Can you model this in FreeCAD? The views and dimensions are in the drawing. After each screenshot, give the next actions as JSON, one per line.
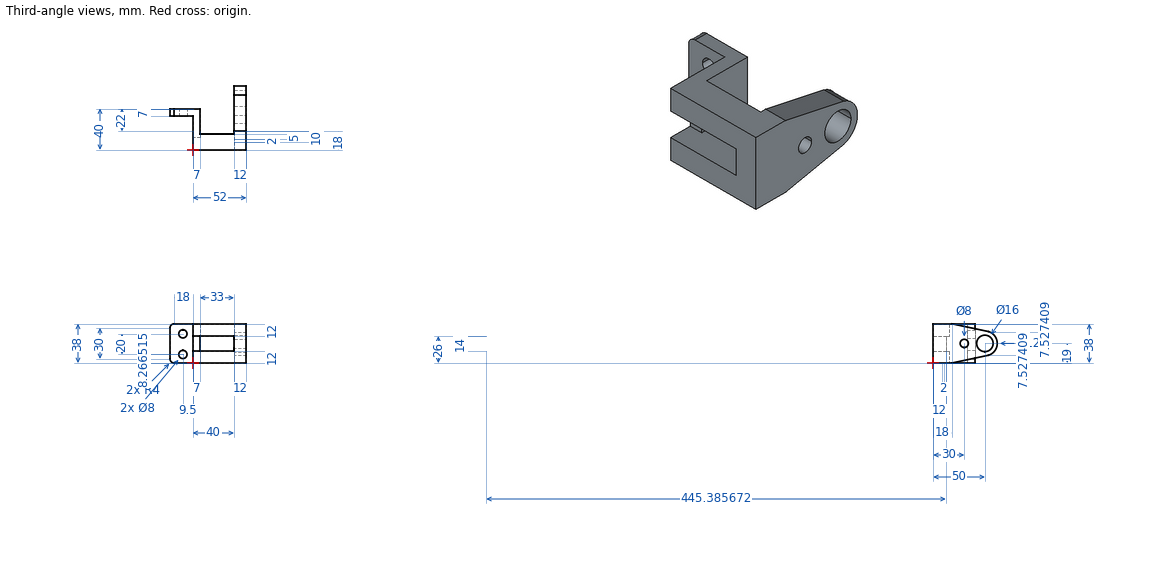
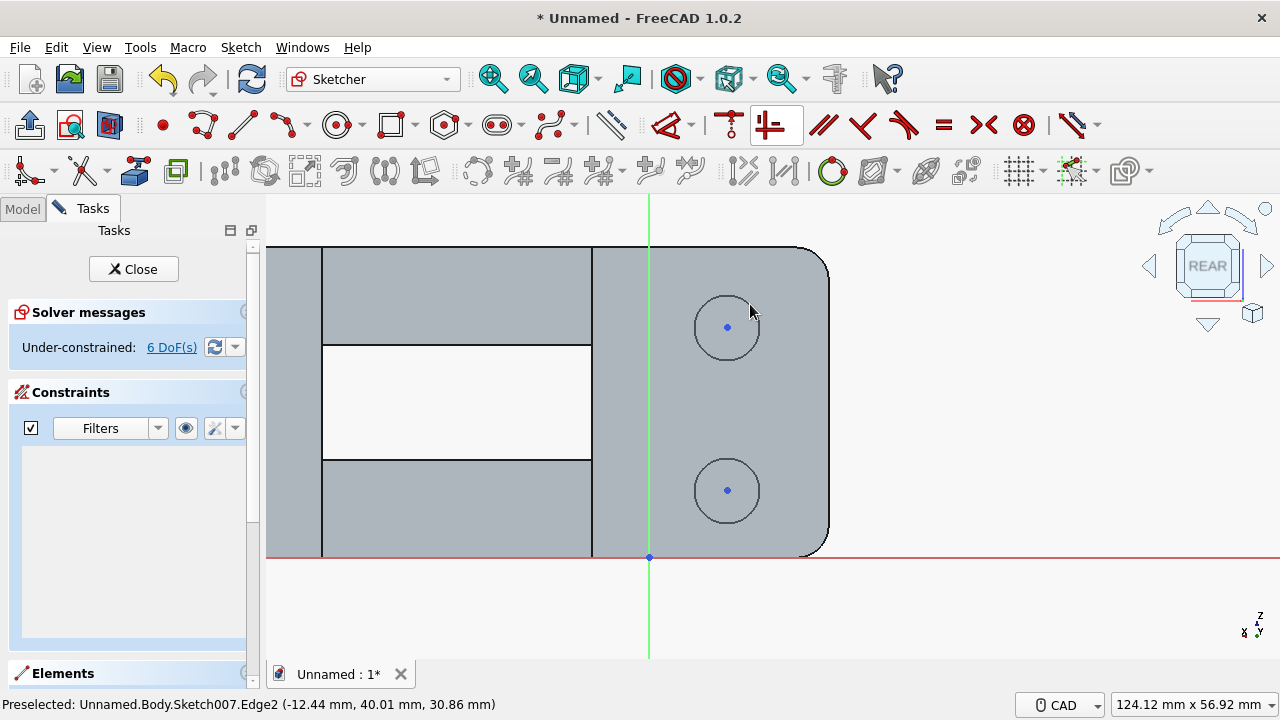
{"action": "left_click", "coordinate": [750, 468]}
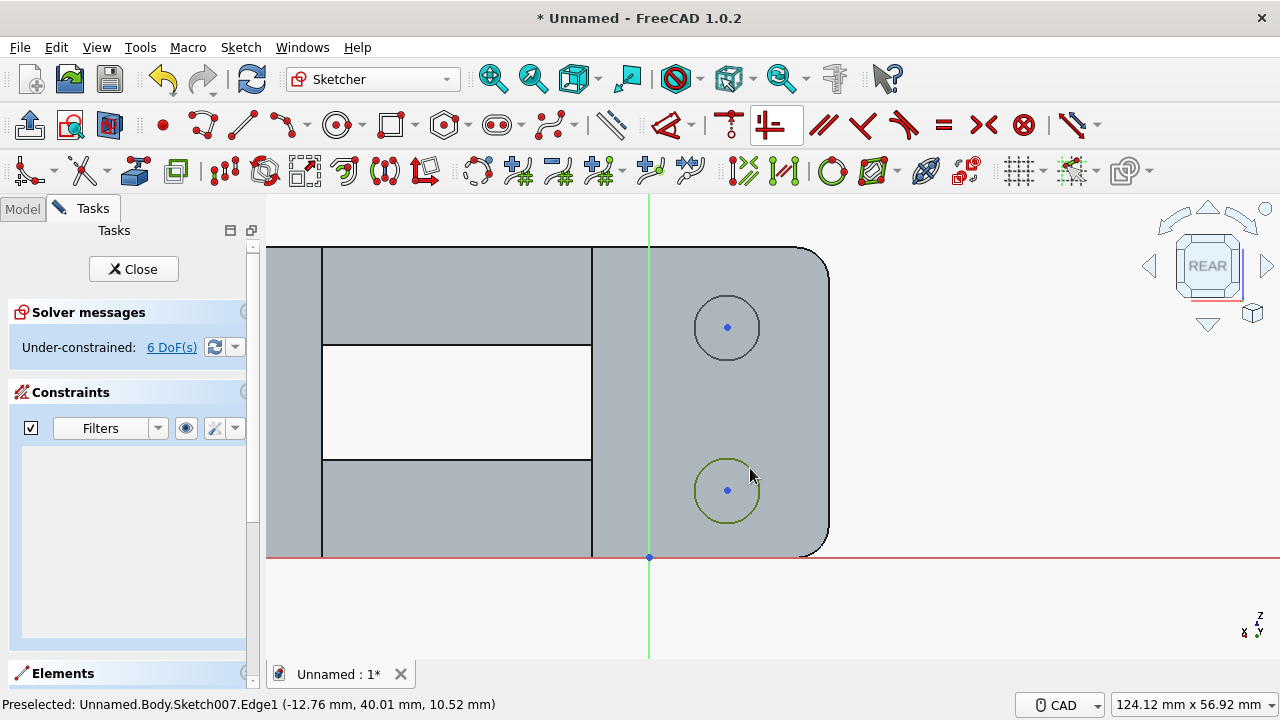
{"action": "left_click", "coordinate": [750, 305]}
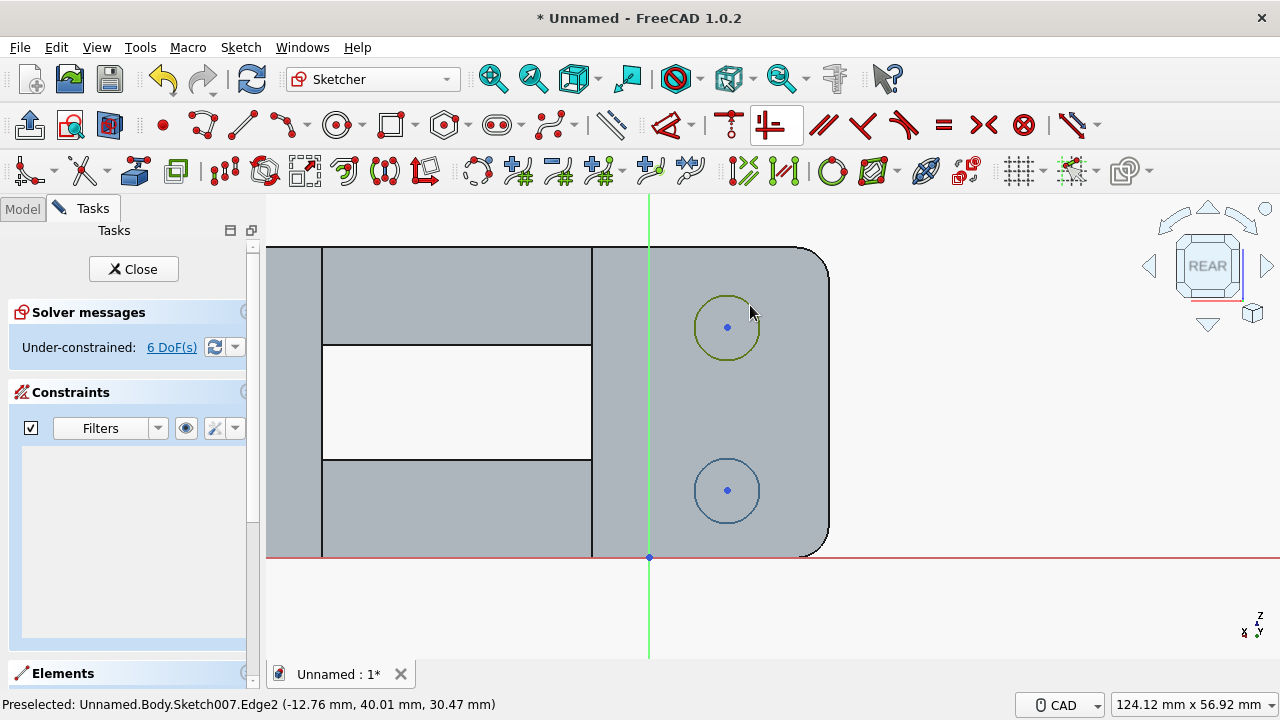
{"action": "left_click", "coordinate": [944, 126]}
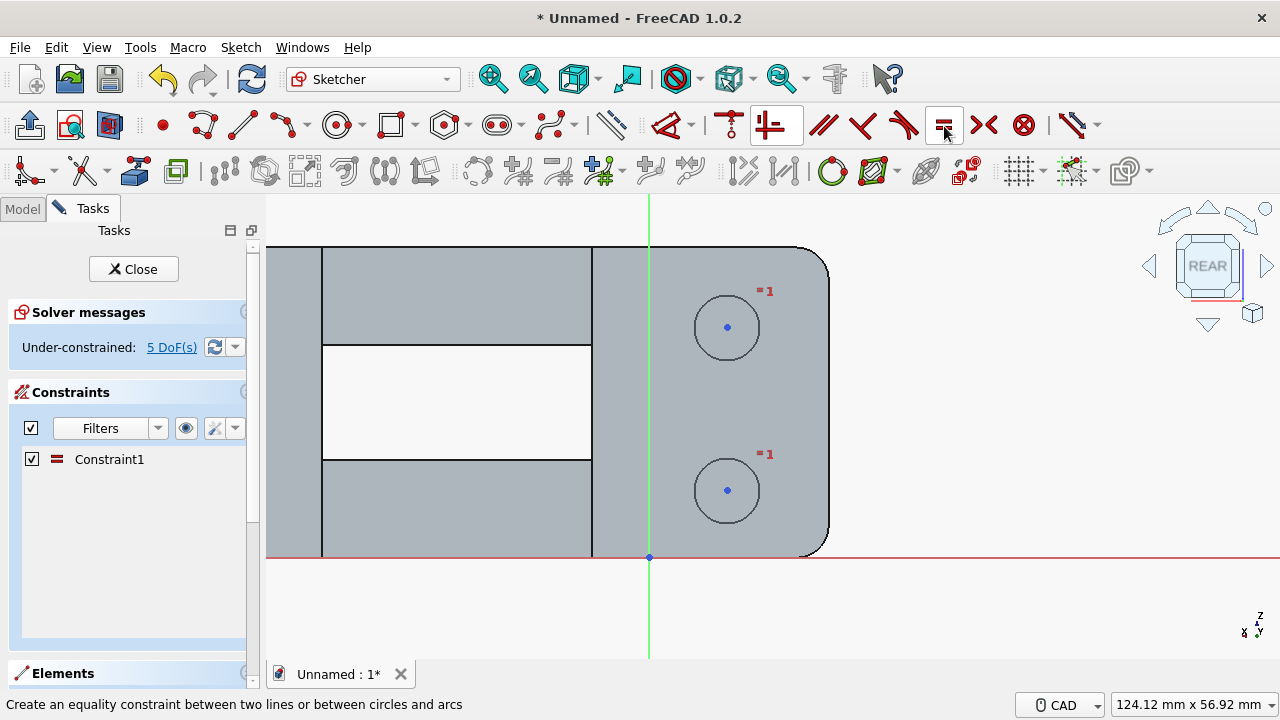
{"action": "left_click", "coordinate": [666, 126]}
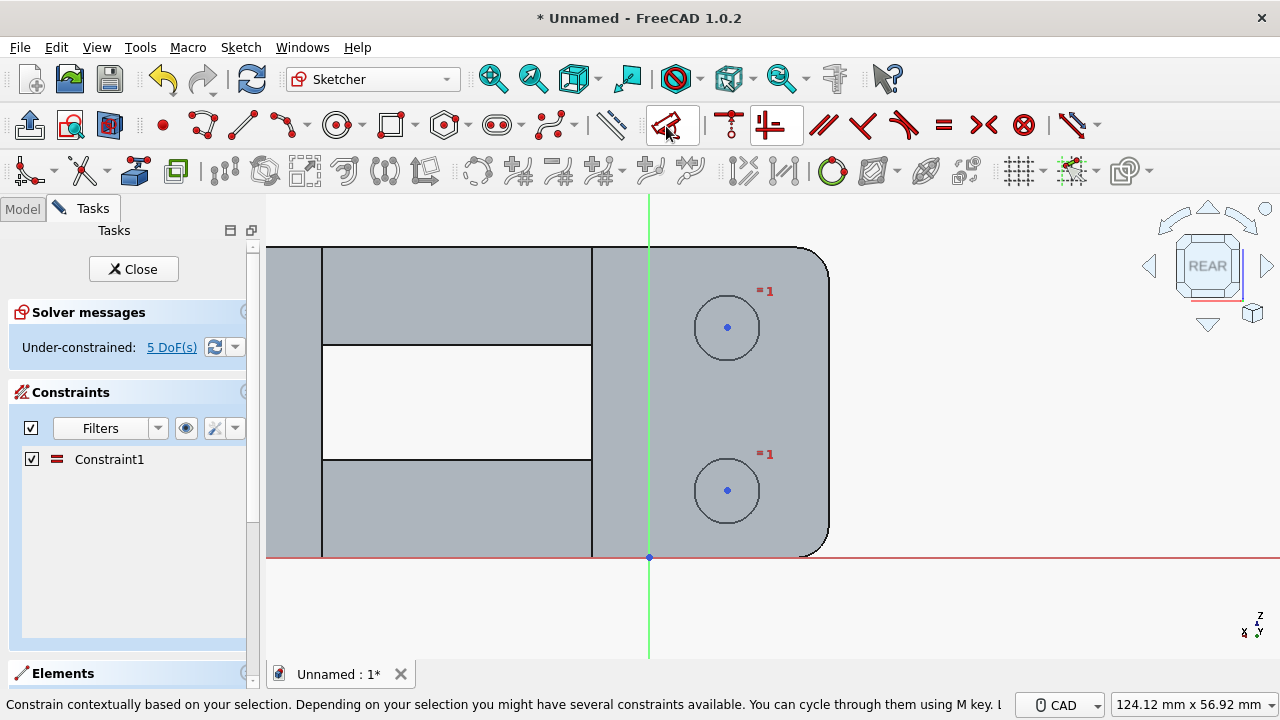
{"action": "left_click", "coordinate": [750, 468]}
{"action": "left_click", "coordinate": [773, 445]}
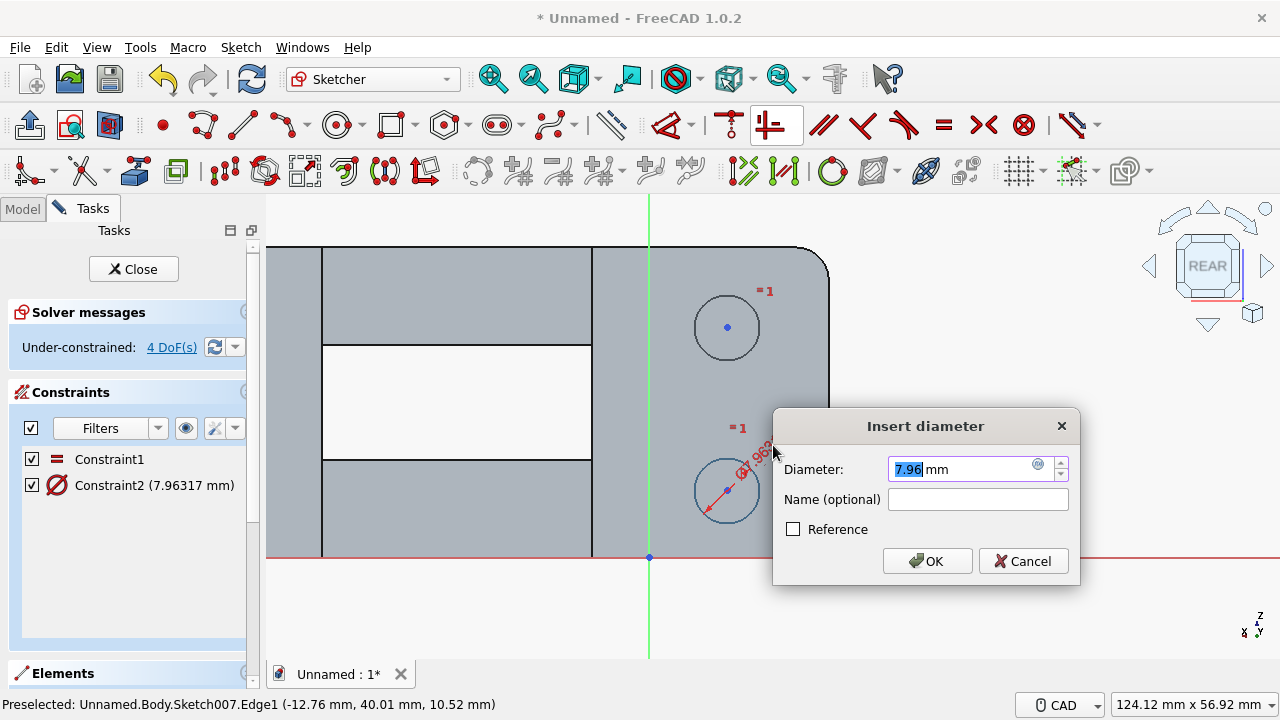
{"action": "type", "text": "8"}
{"action": "key", "text": "Return"}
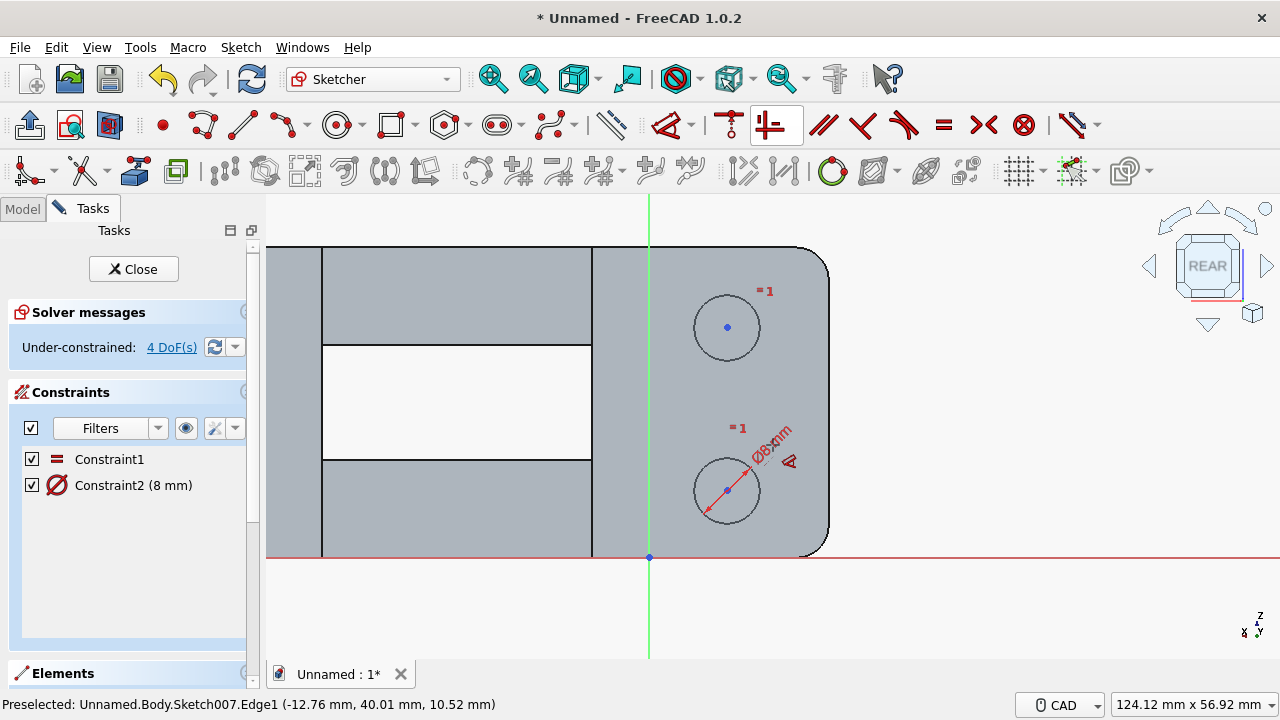
{"action": "left_click", "coordinate": [727, 491]}
{"action": "left_click", "coordinate": [688, 592]}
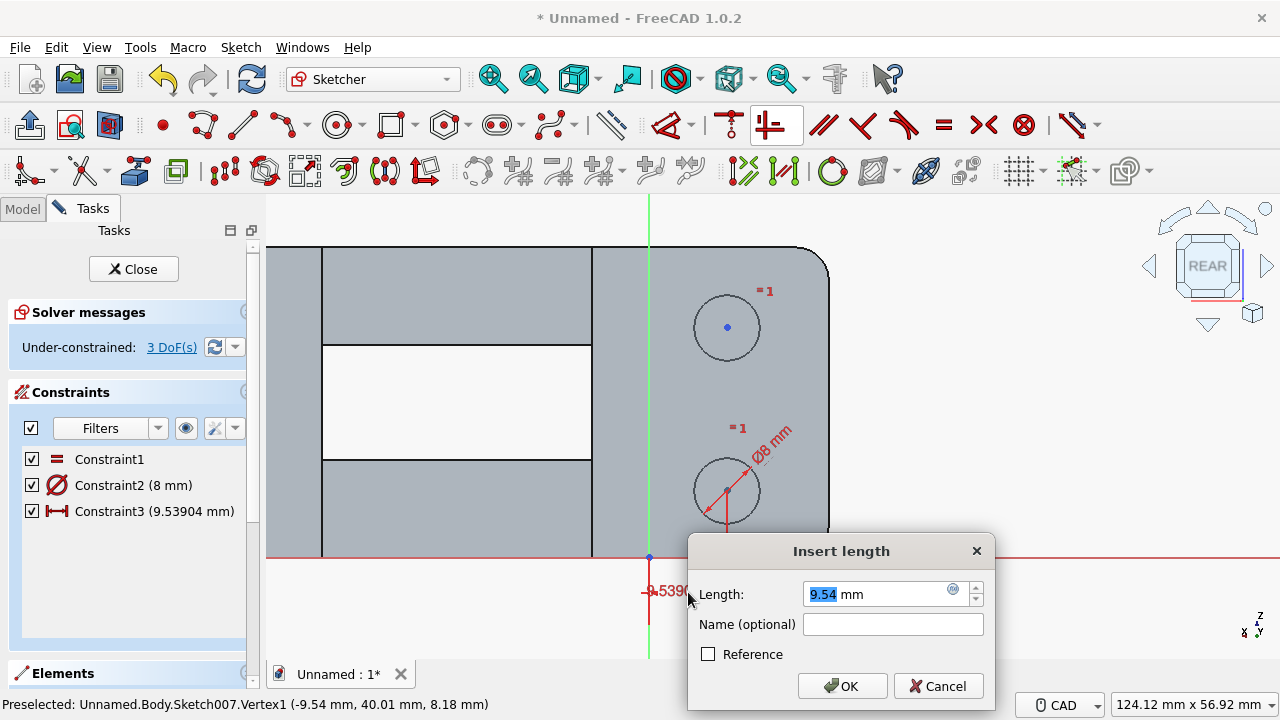
{"action": "type", "text": "9.5"}
{"action": "key", "text": "Return"}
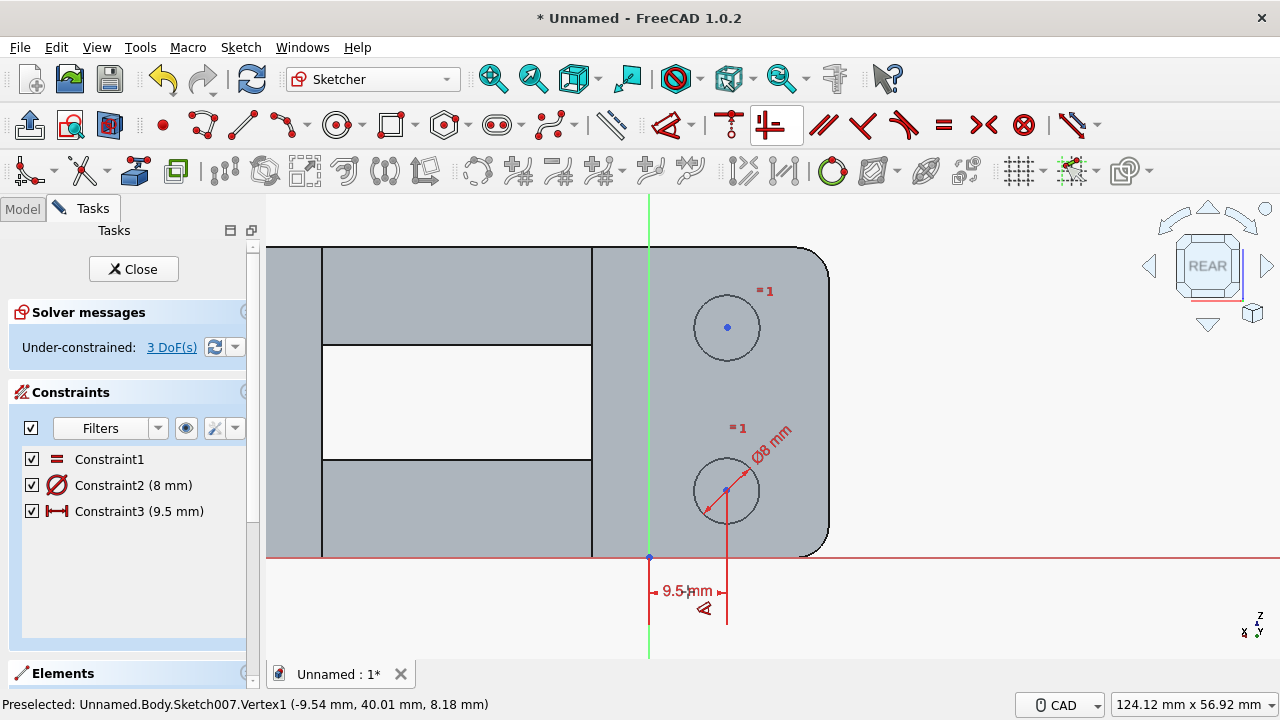
{"action": "left_click", "coordinate": [727, 328]}
{"action": "left_click", "coordinate": [688, 294]}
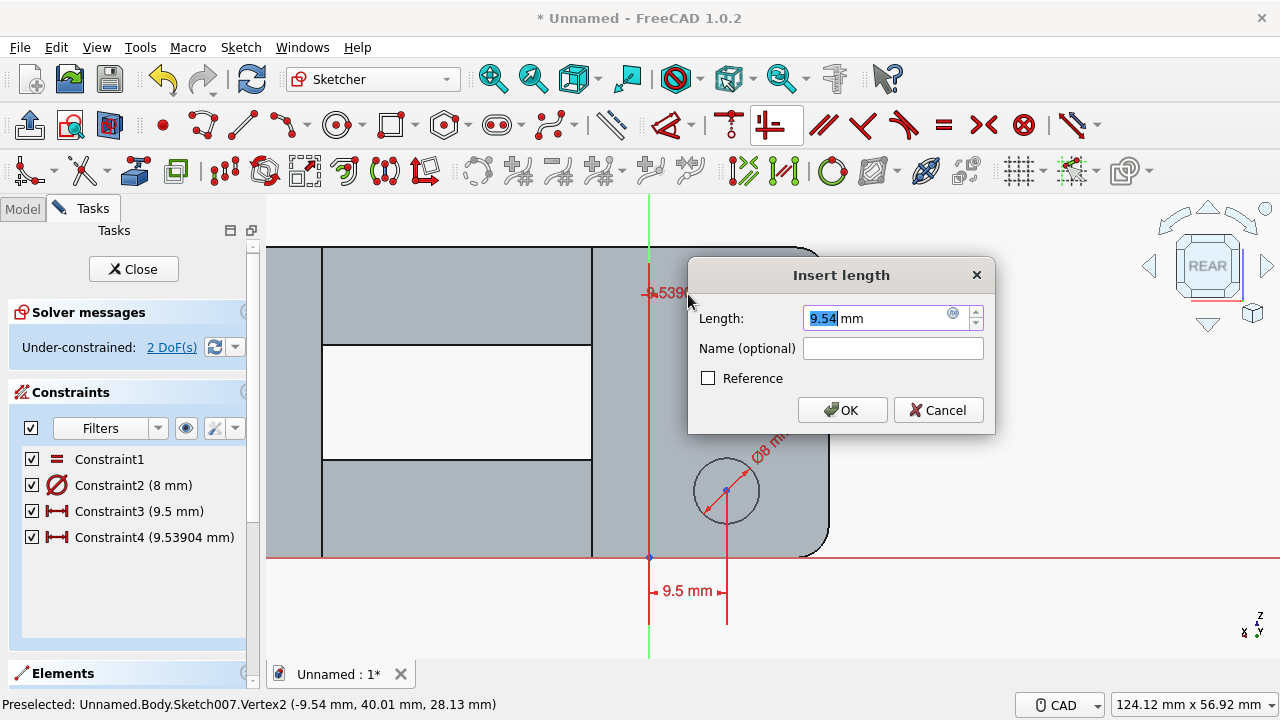
{"action": "type", "text": "9.5"}
{"action": "key", "text": "Return"}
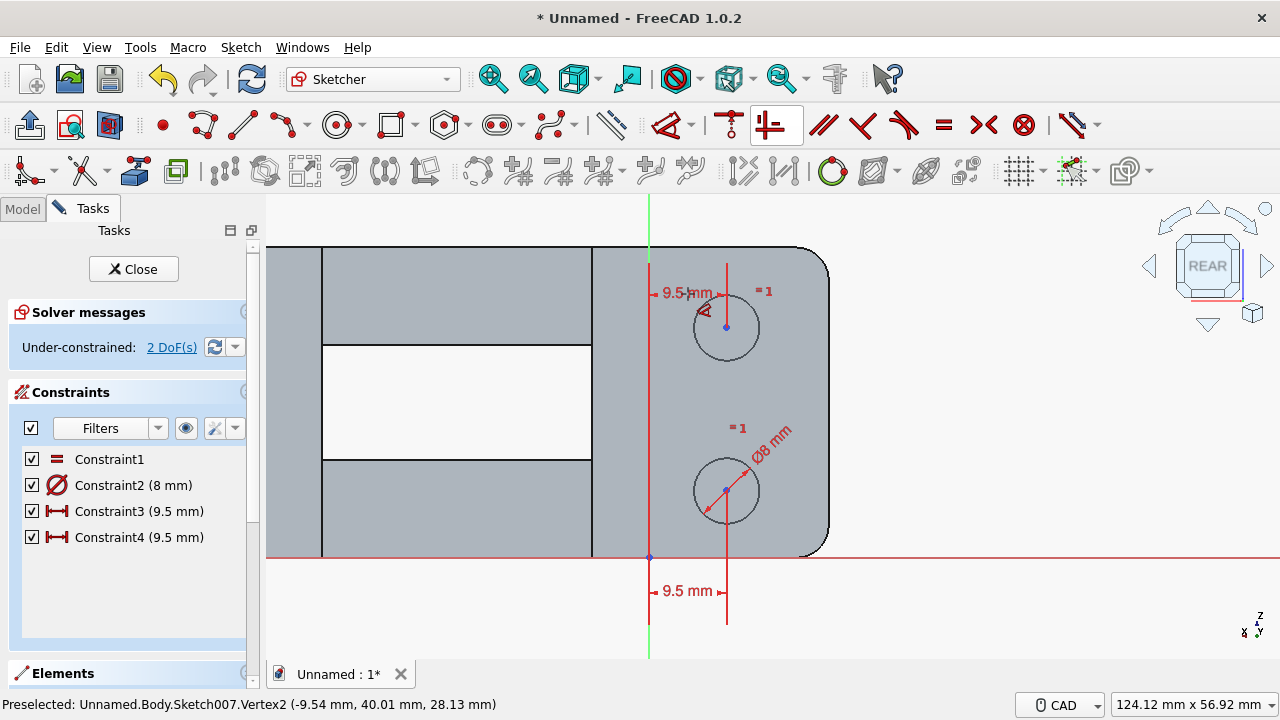
{"action": "left_click", "coordinate": [727, 491]}